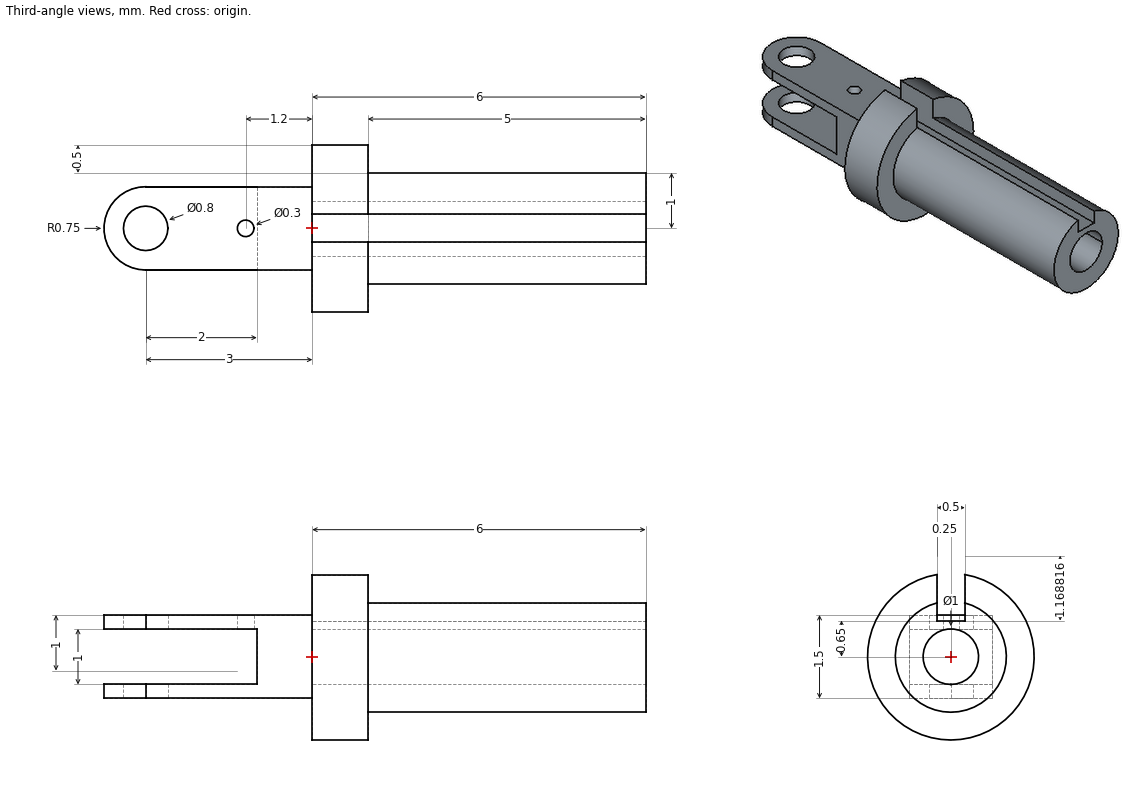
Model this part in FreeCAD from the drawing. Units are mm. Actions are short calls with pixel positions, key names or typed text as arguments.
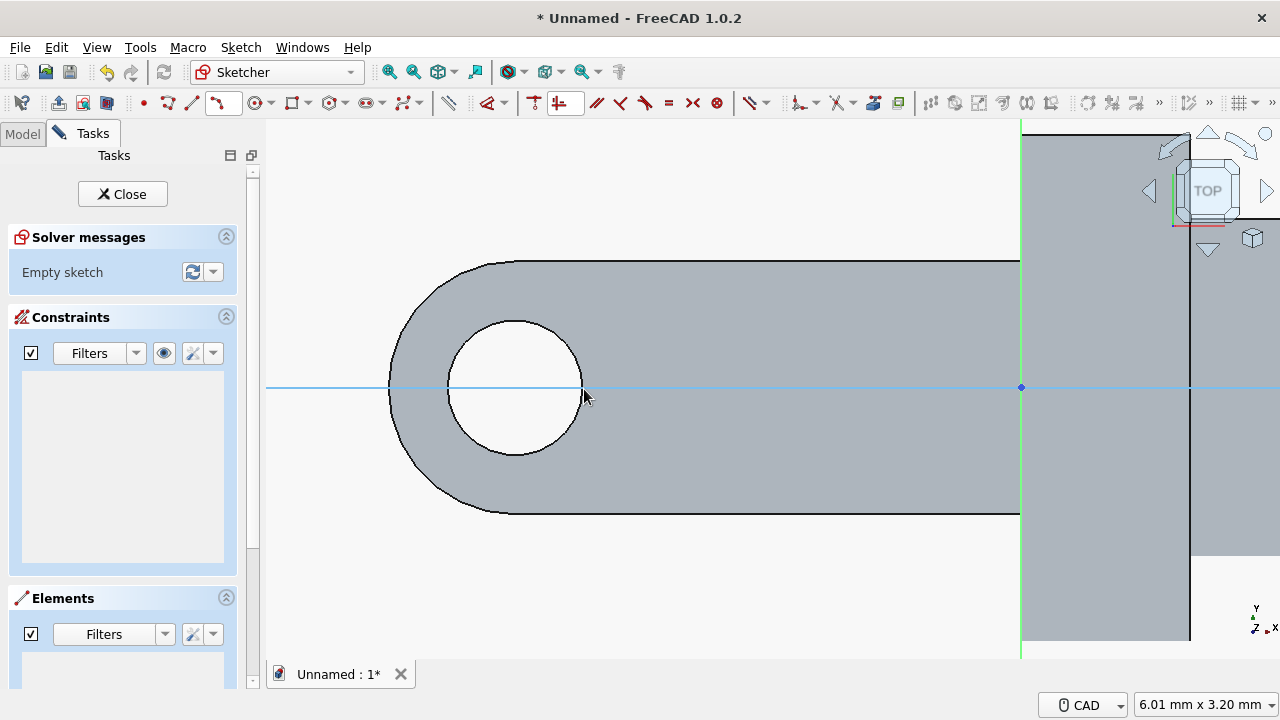
click(168, 104)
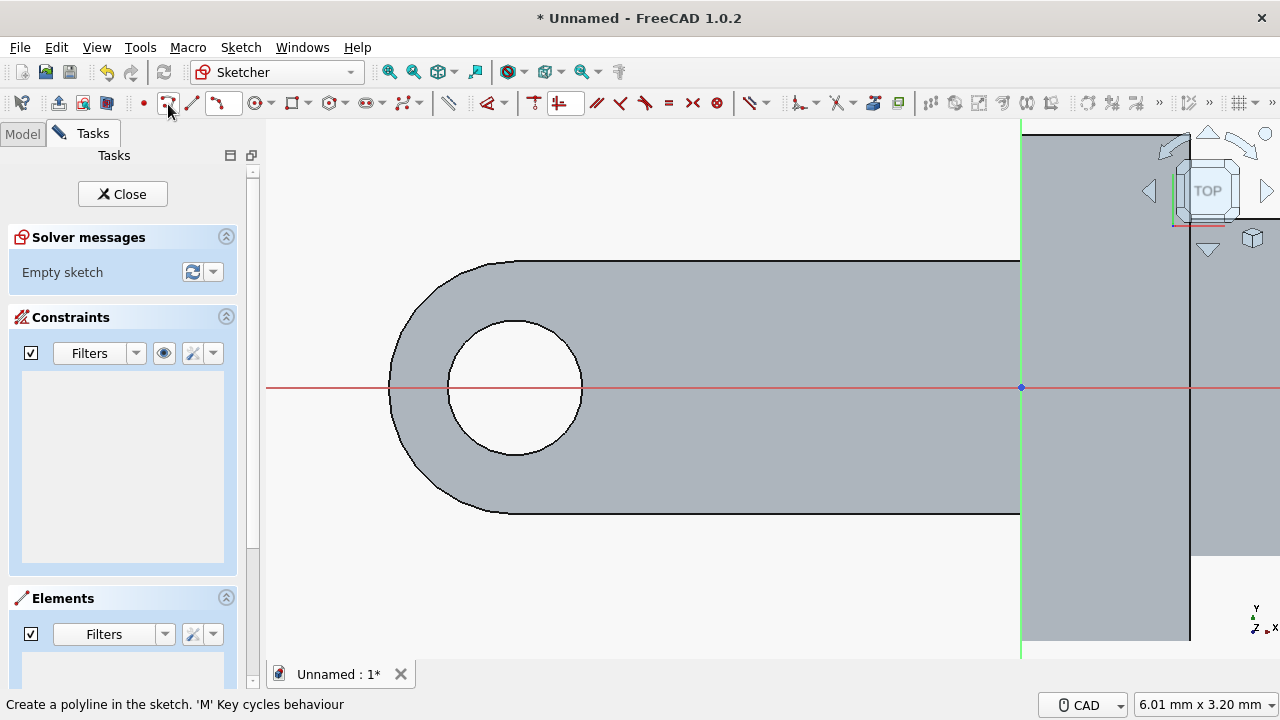
click(515, 514)
click(852, 514)
click(852, 261)
click(515, 261)
right_click(515, 261)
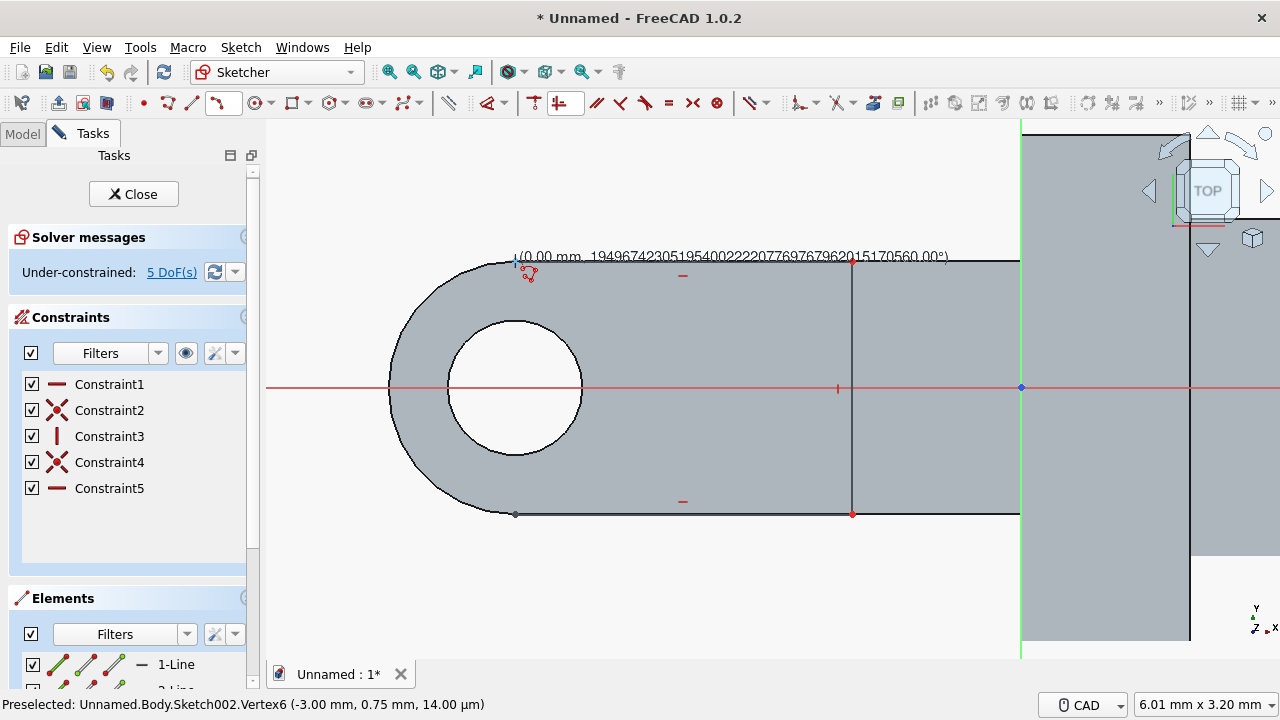
click(218, 104)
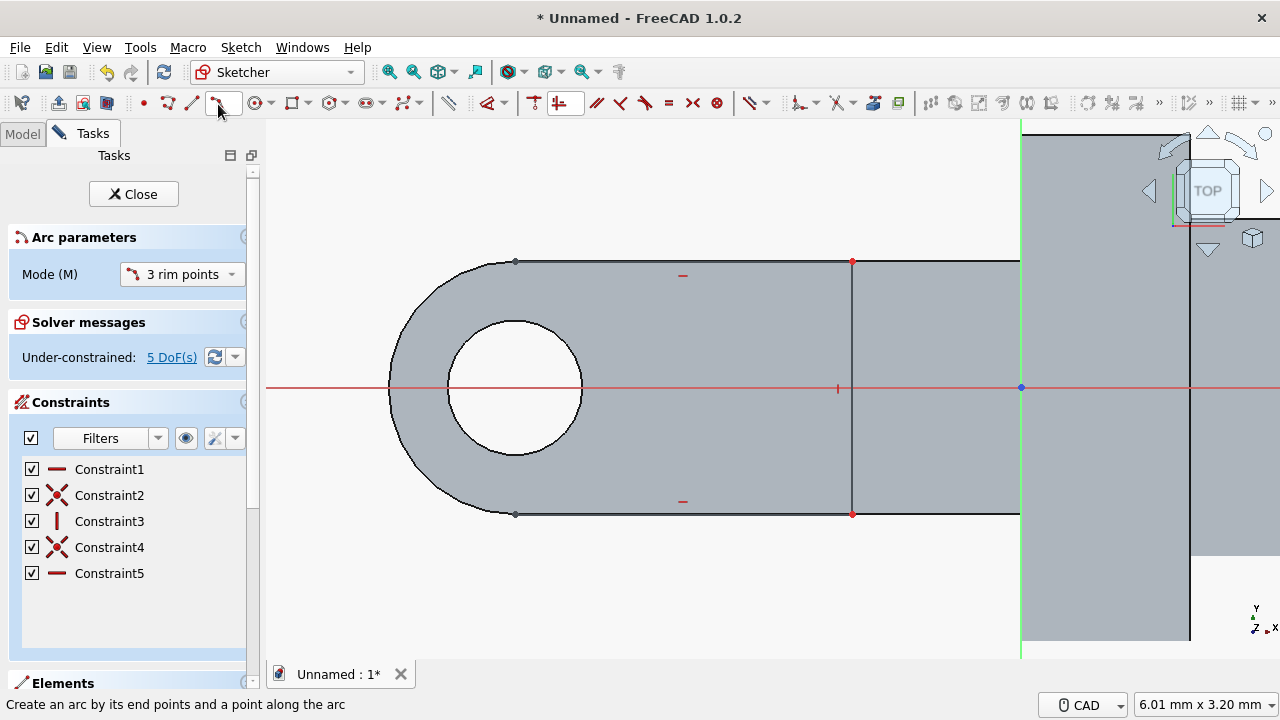
click(515, 262)
click(515, 515)
click(395, 349)
key(Escape)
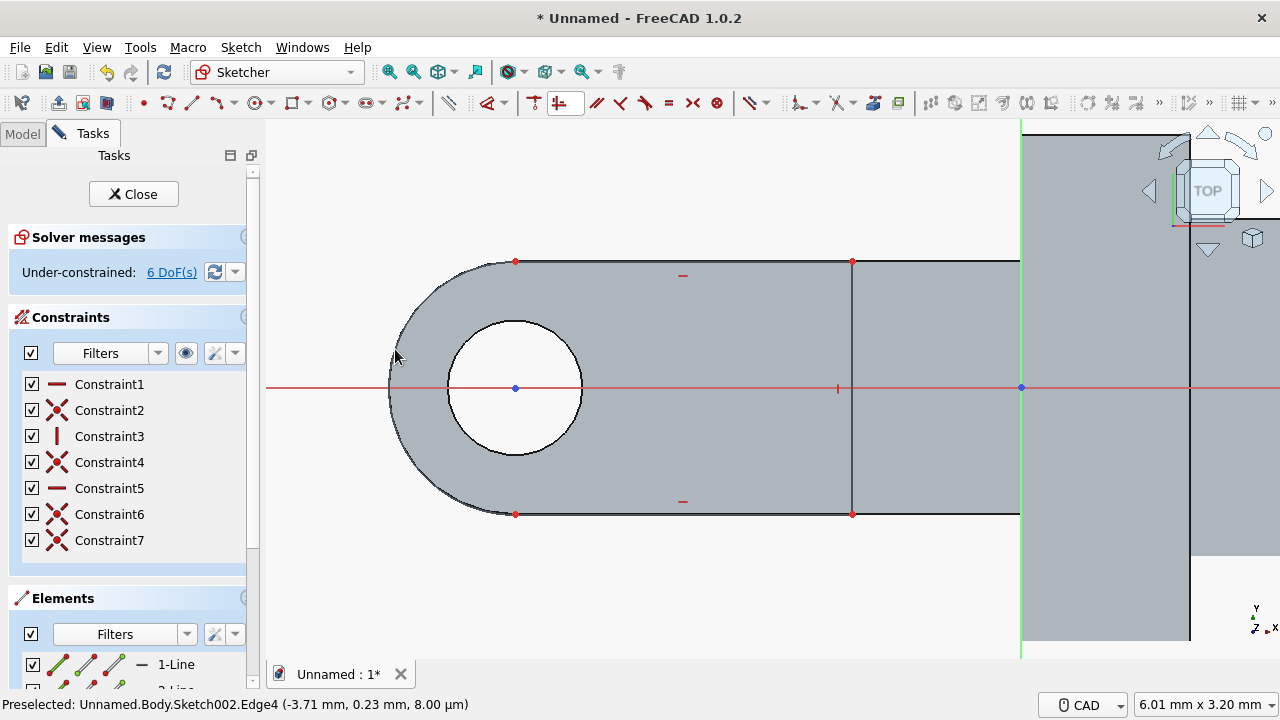
click(616, 515)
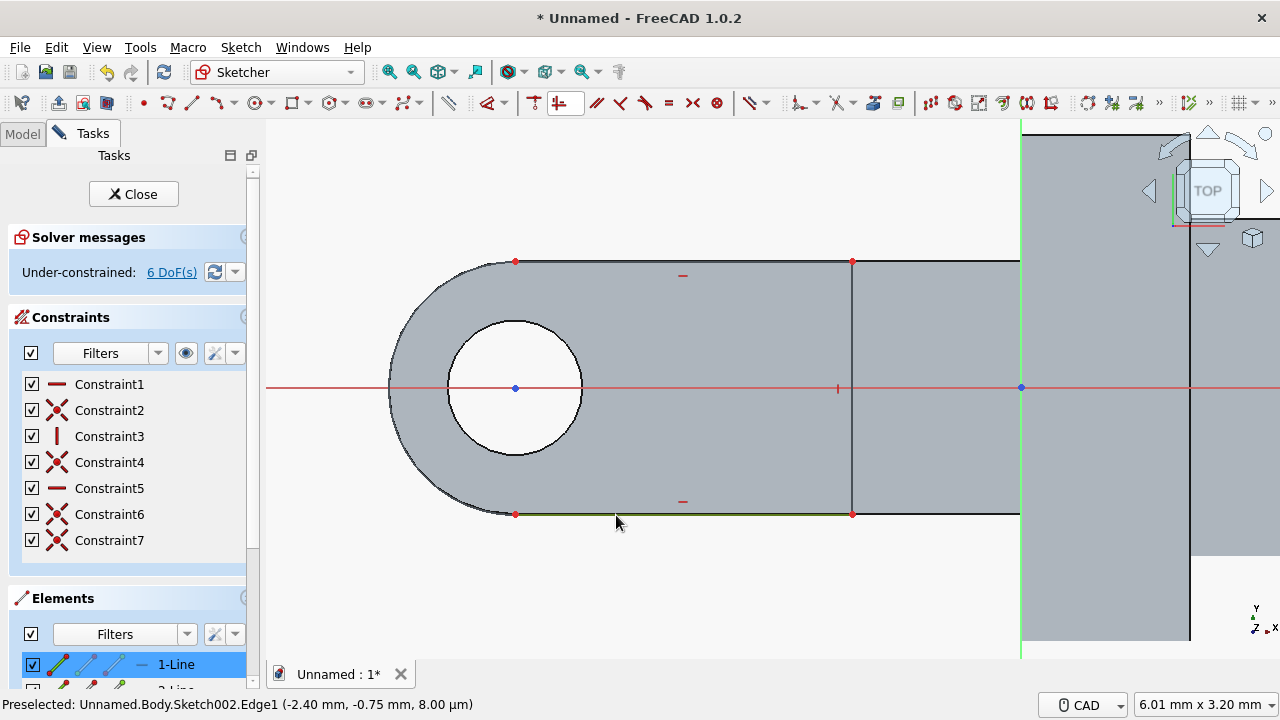
click(413, 314)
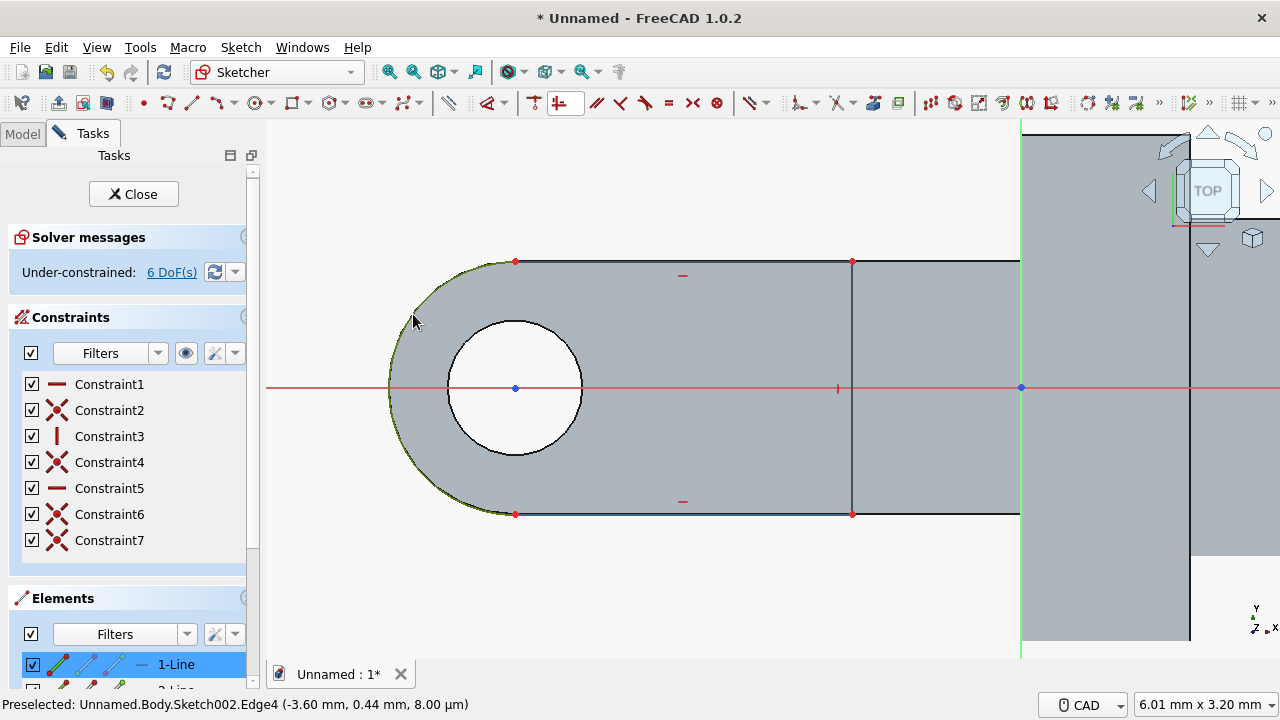
click(646, 104)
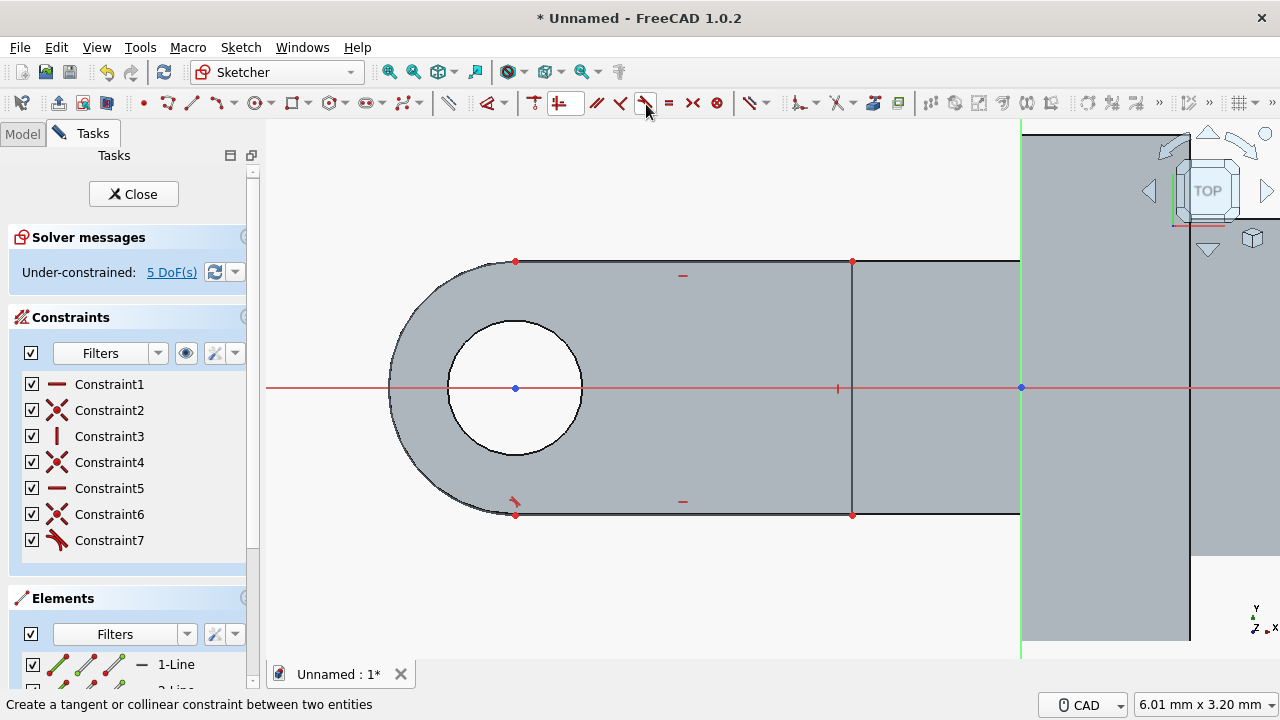
click(751, 262)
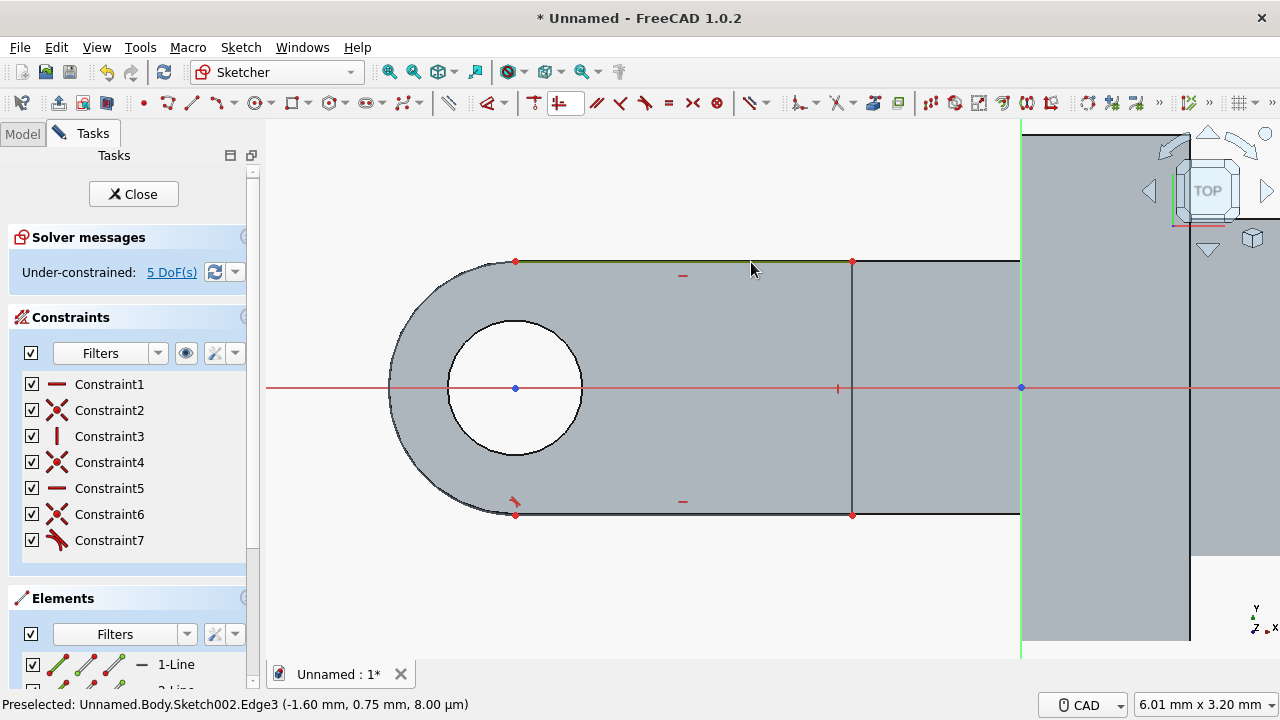
click(413, 314)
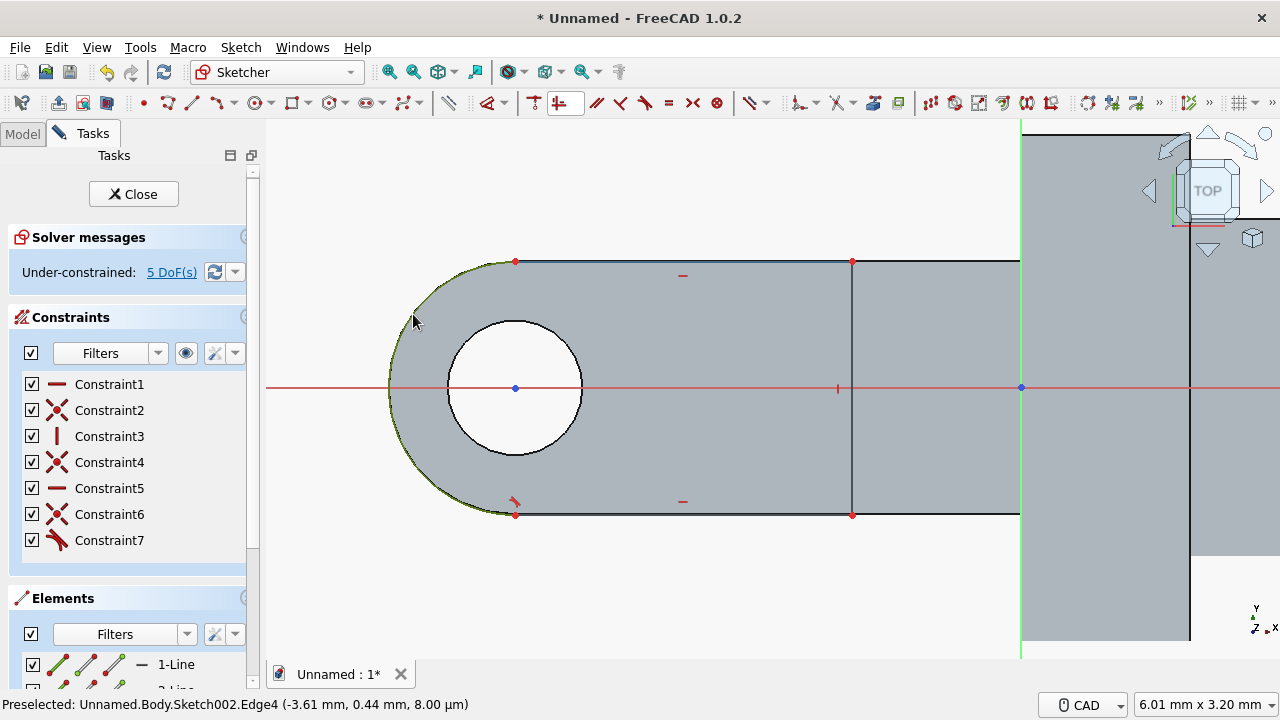
click(646, 104)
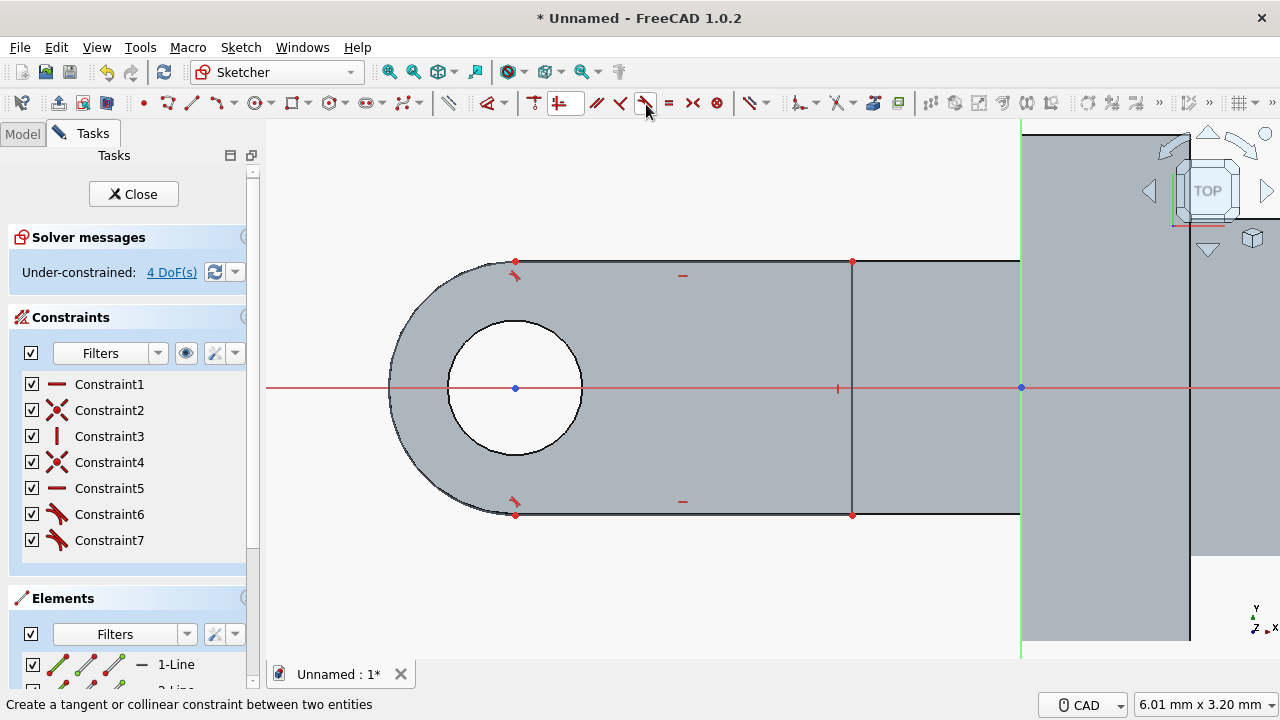
click(516, 389)